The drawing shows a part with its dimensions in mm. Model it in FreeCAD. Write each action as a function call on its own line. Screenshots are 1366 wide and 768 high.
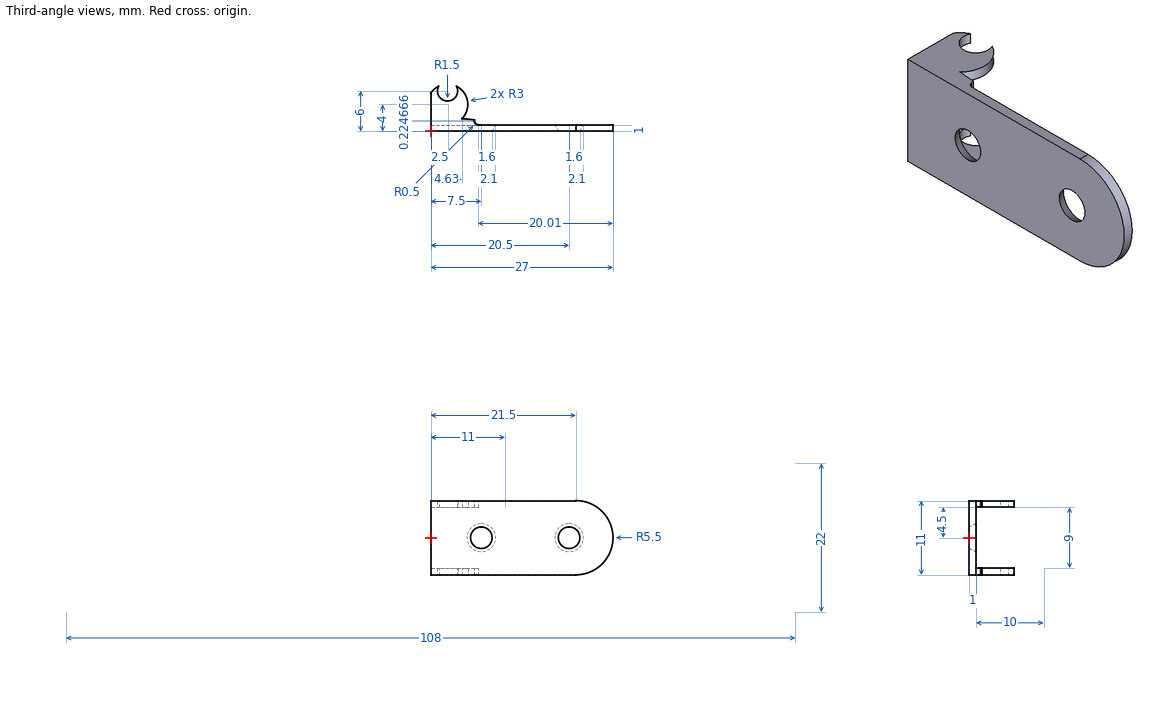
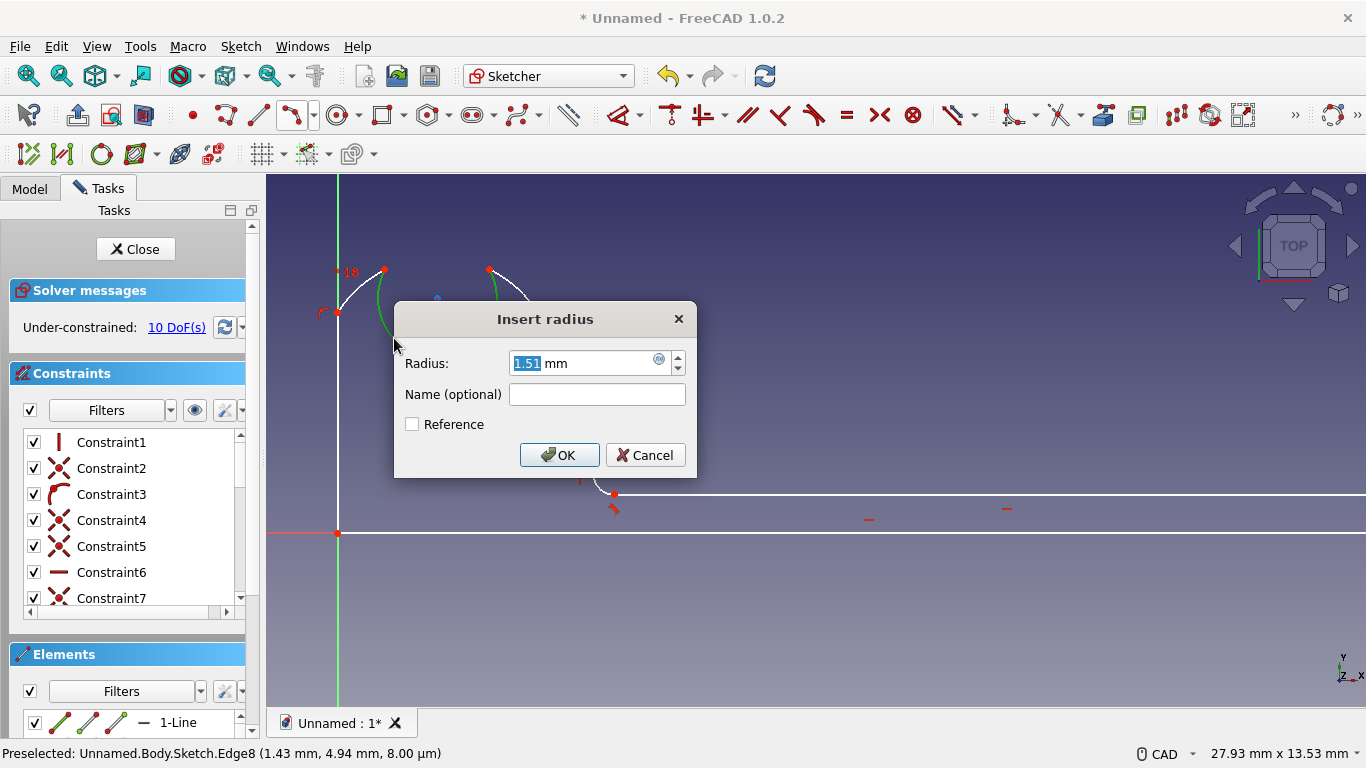
text(1.5)
key(Return)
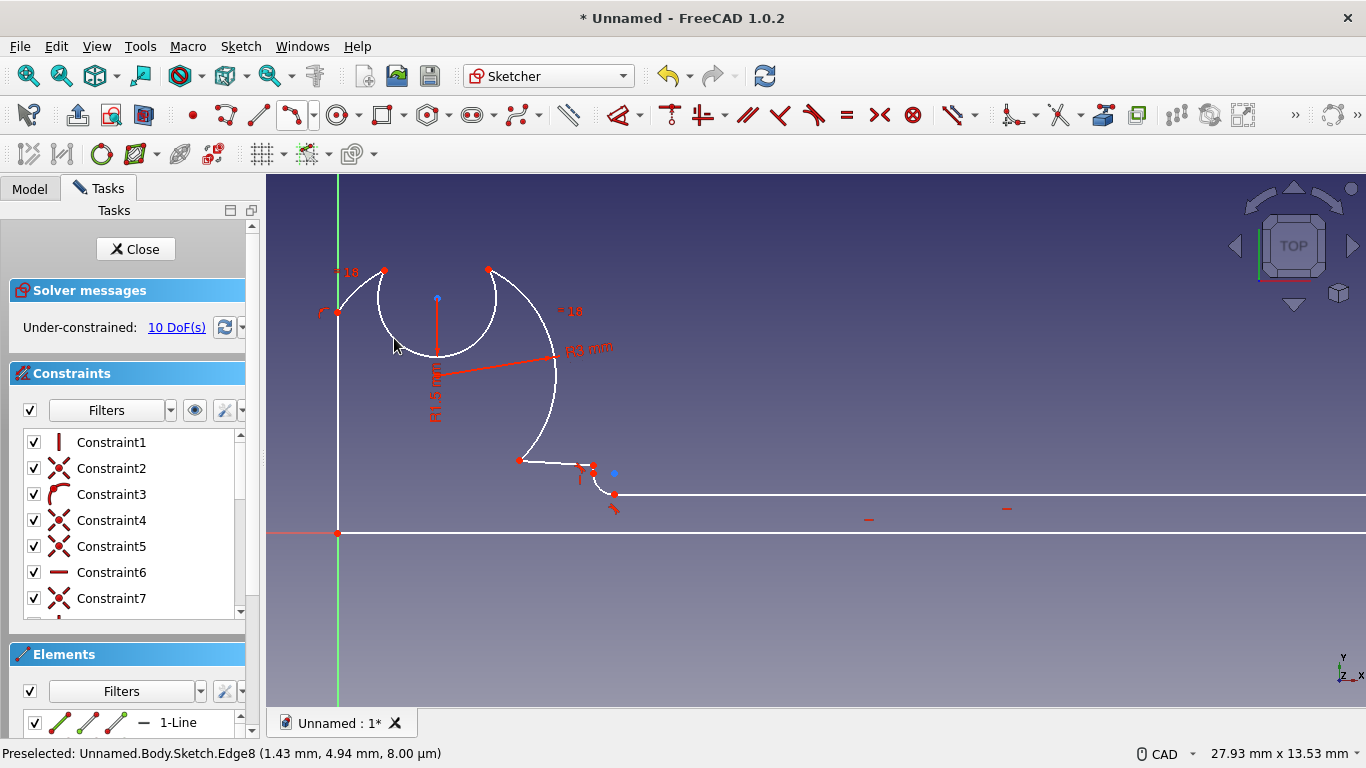
scroll(596, 483, up, 4)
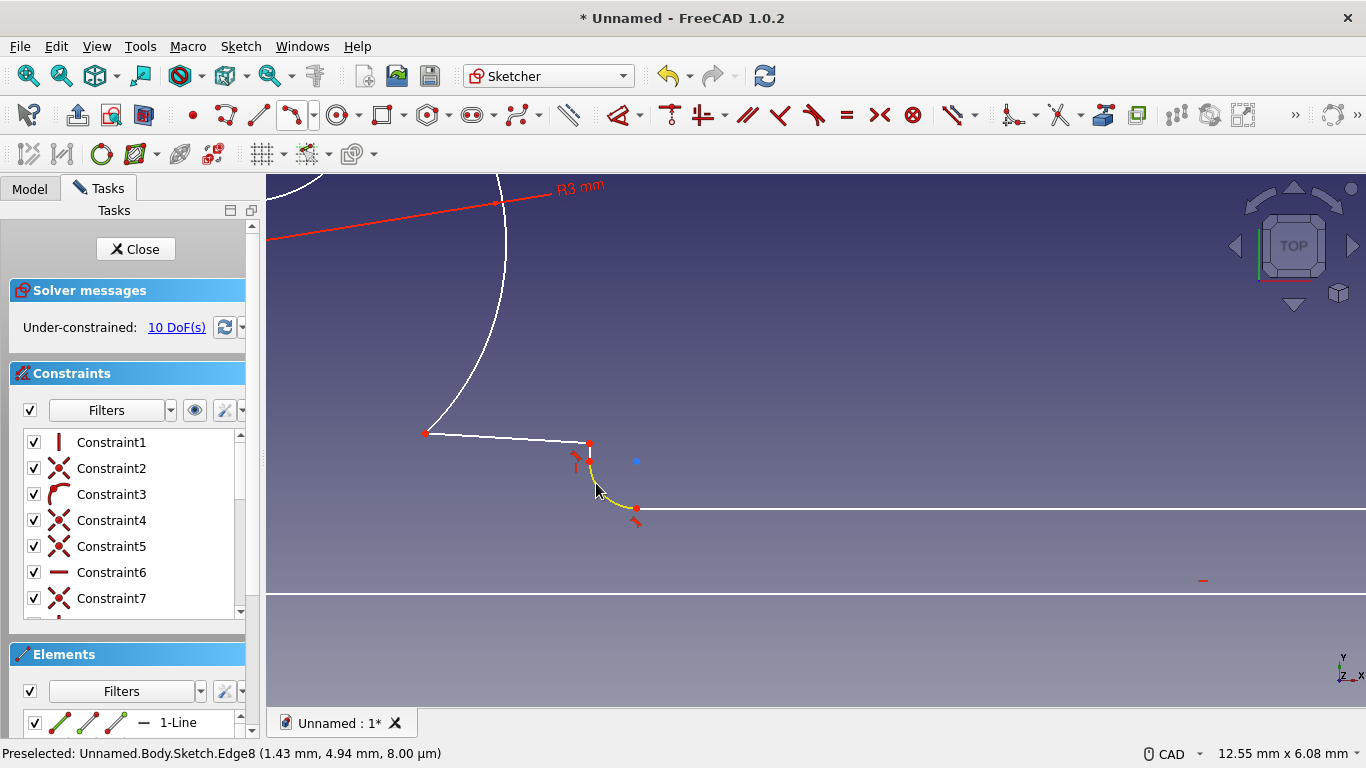
click(595, 483)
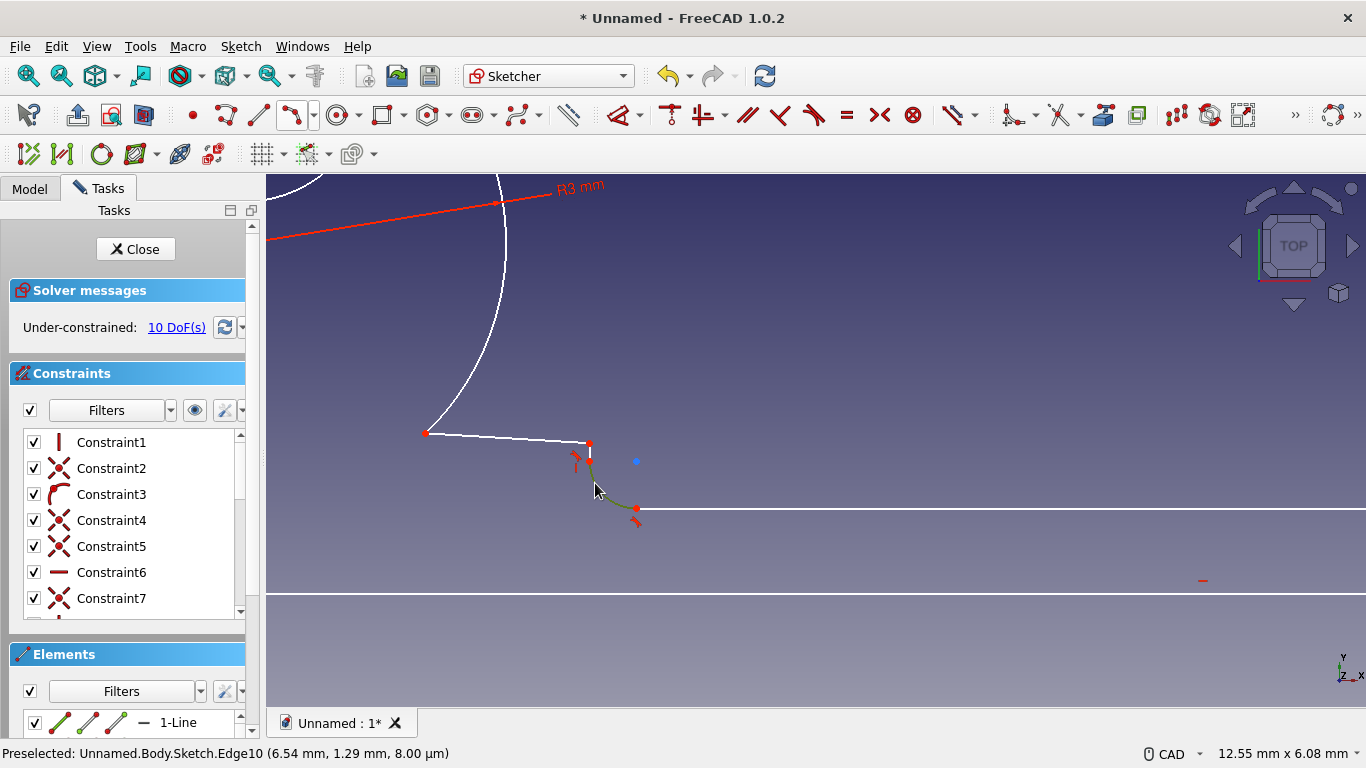
key(k)
key(r)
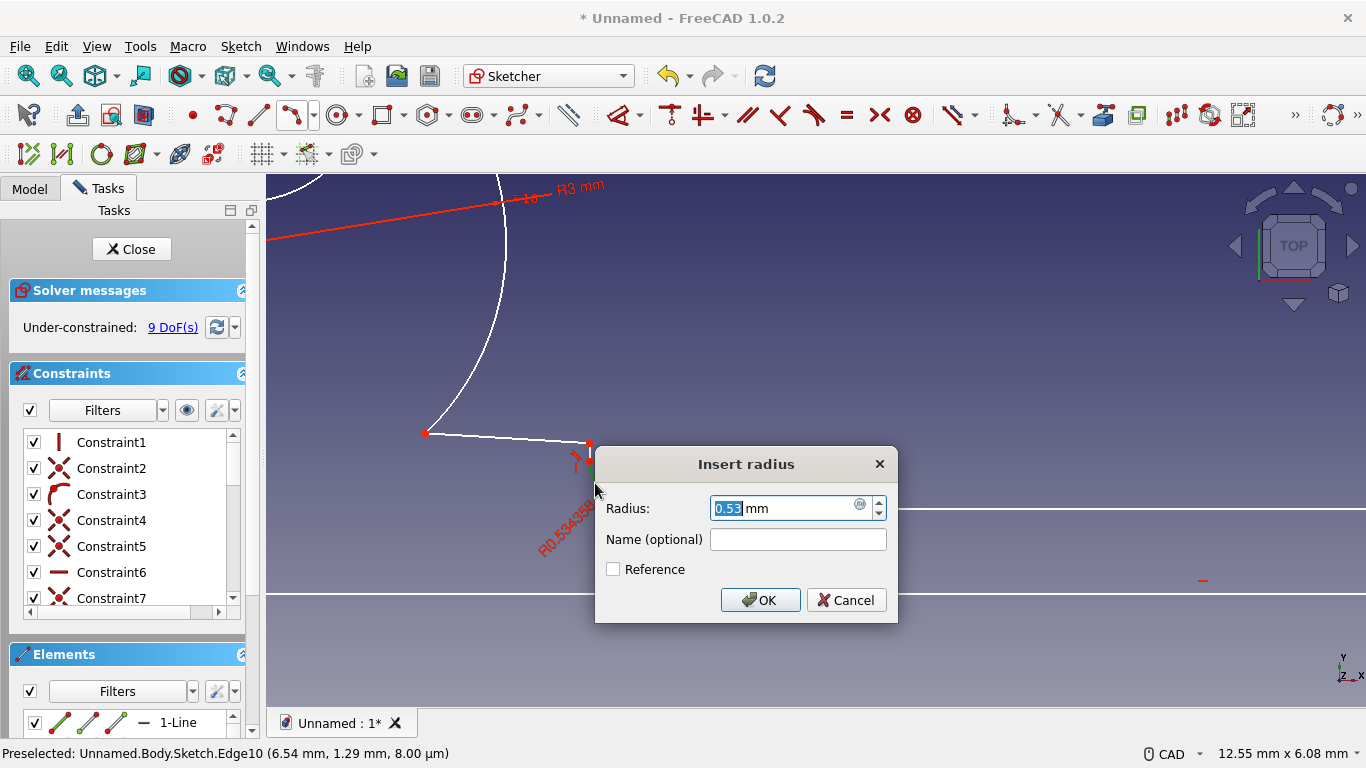
text(0.5)
key(Return)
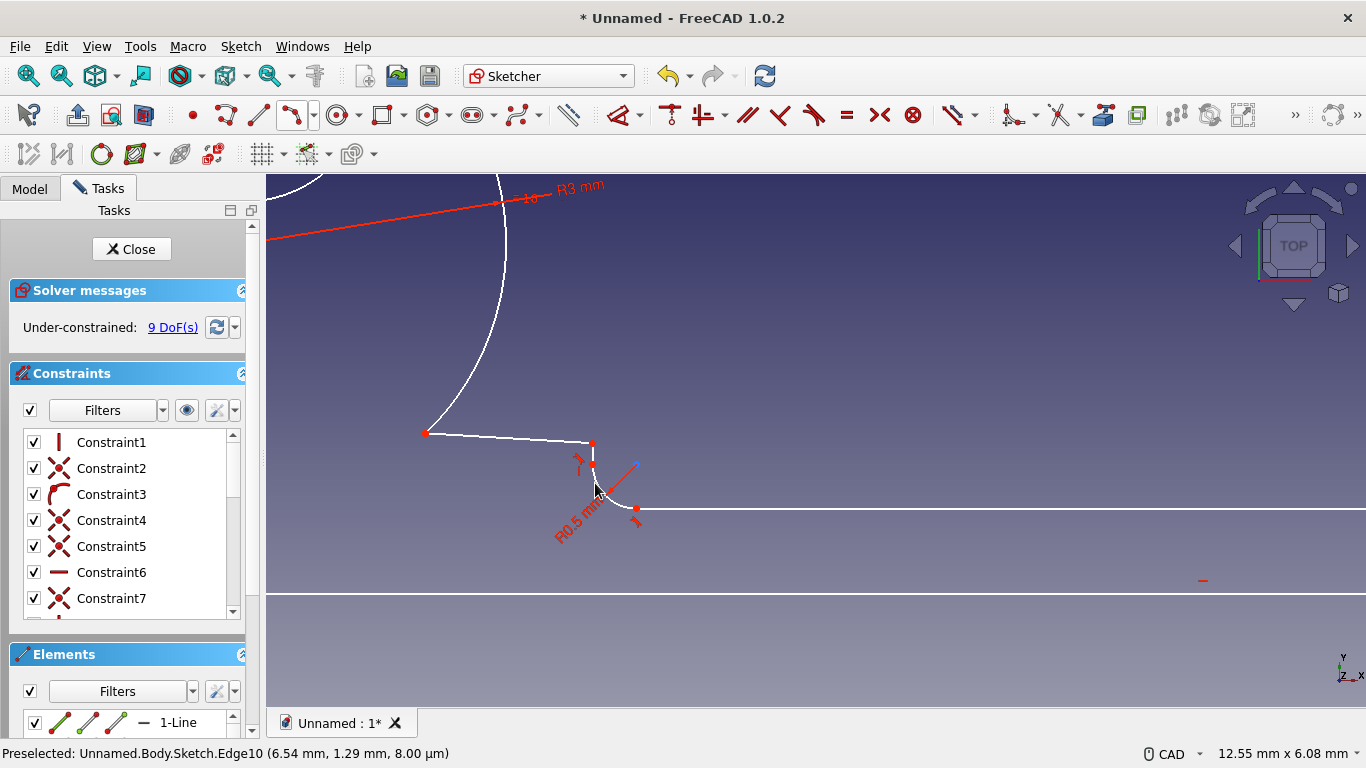
scroll(598, 486, down, 7)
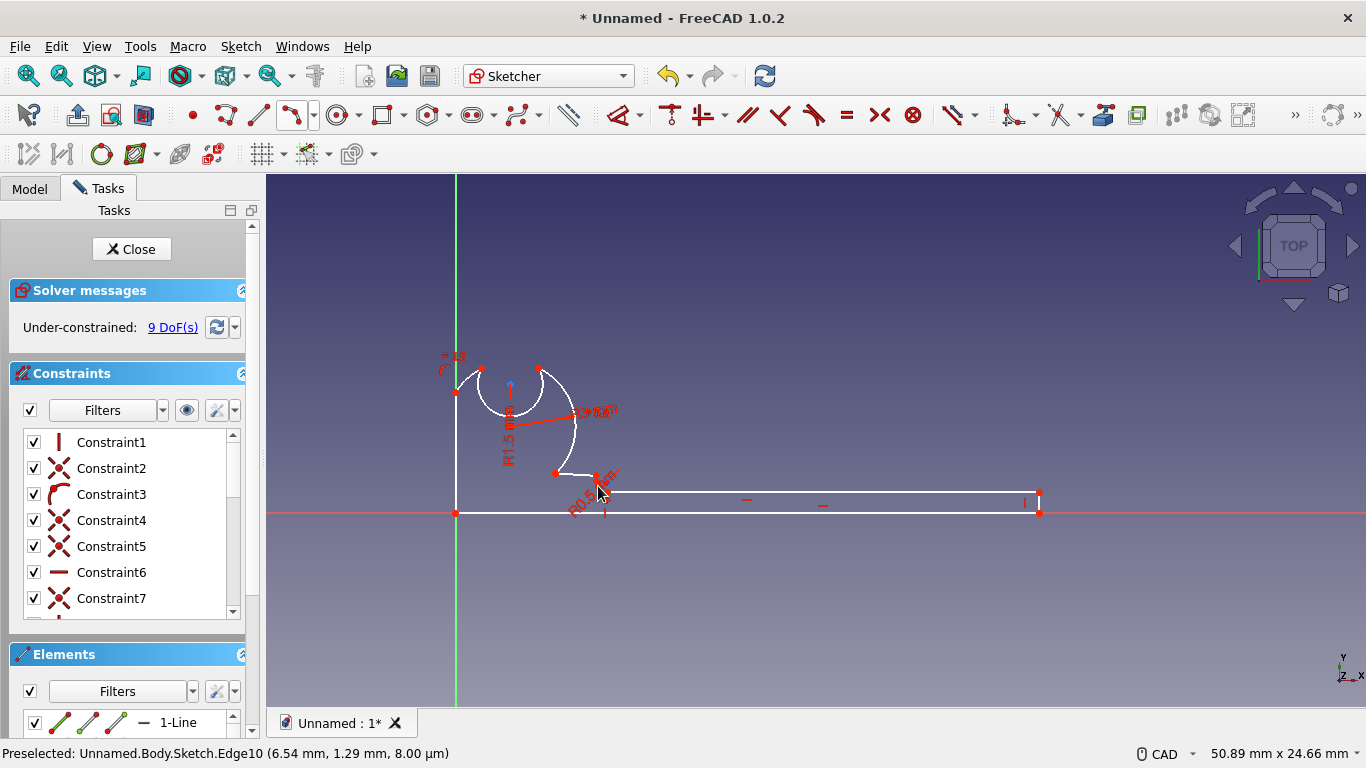
scroll(1039, 507, up, 4)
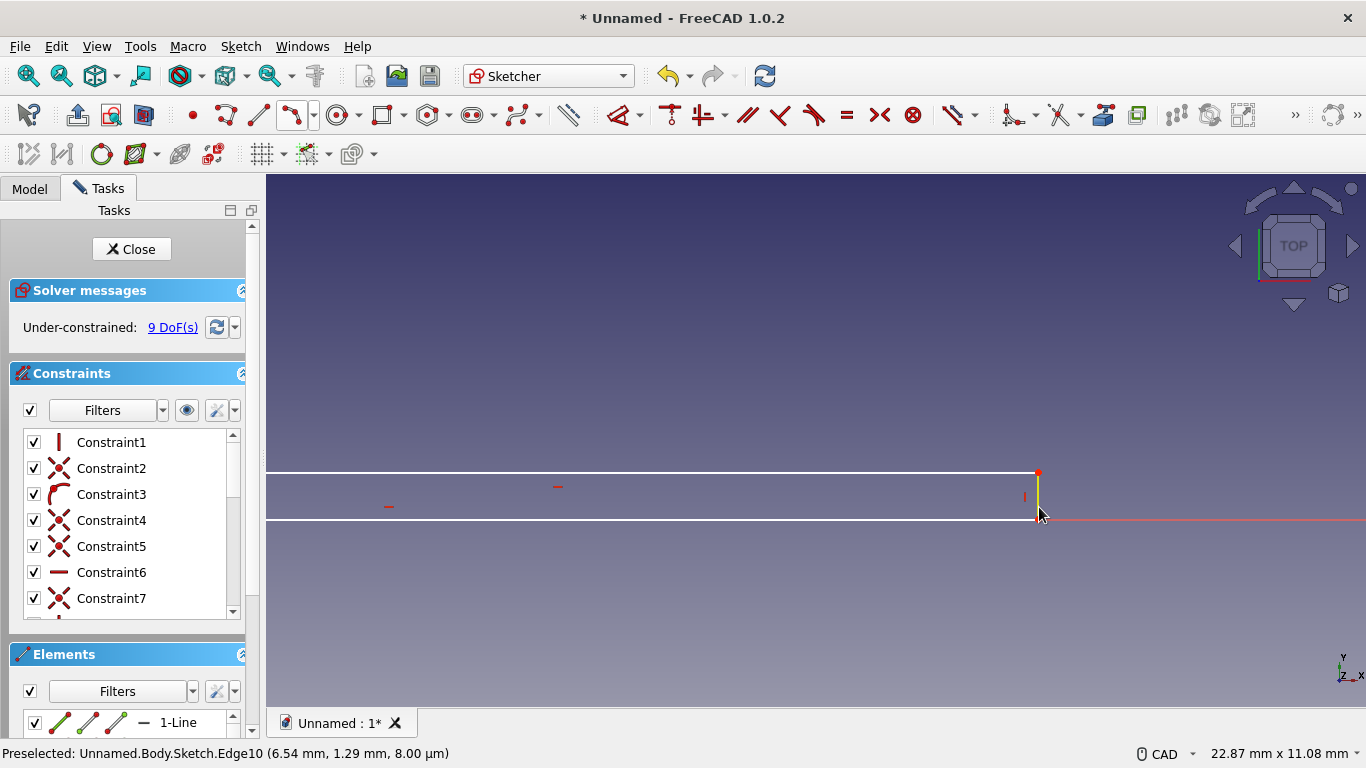
click(1038, 506)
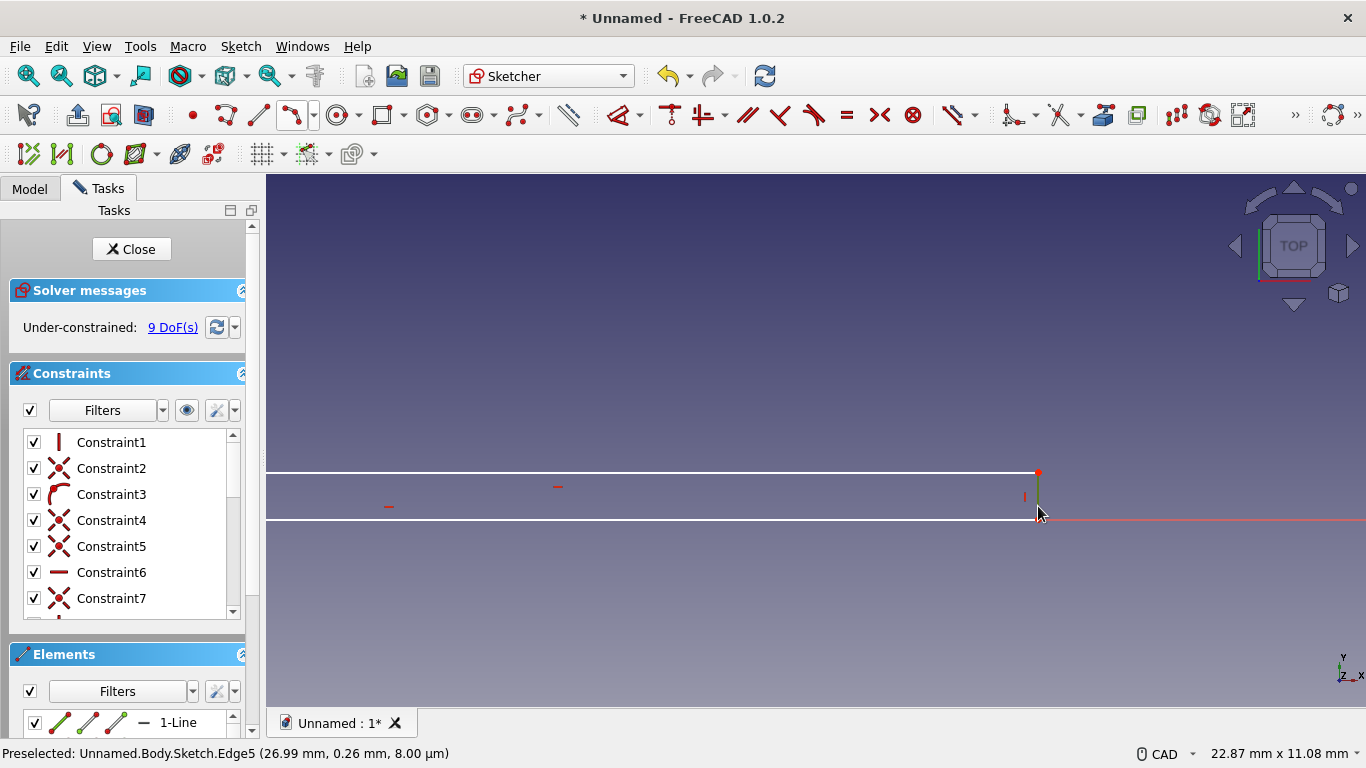
key(i)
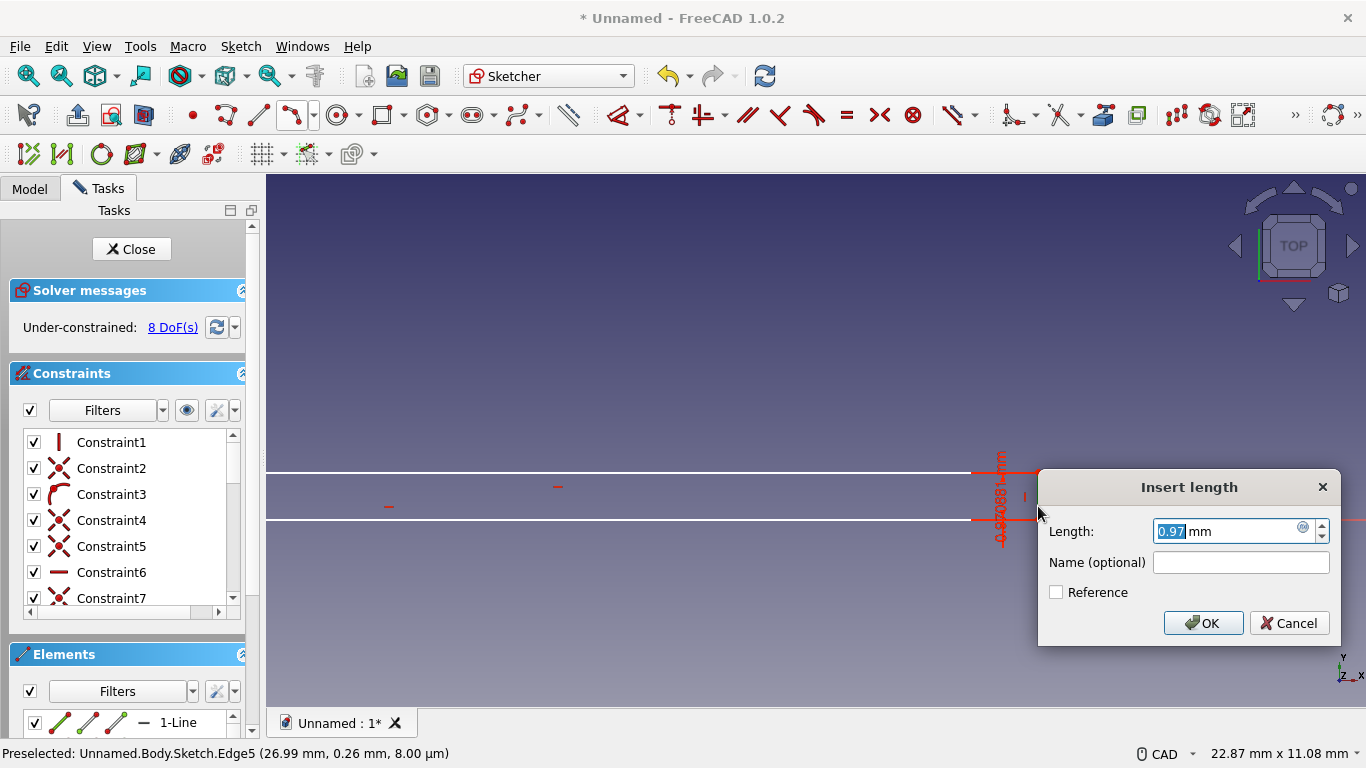
text(1)
key(Return)